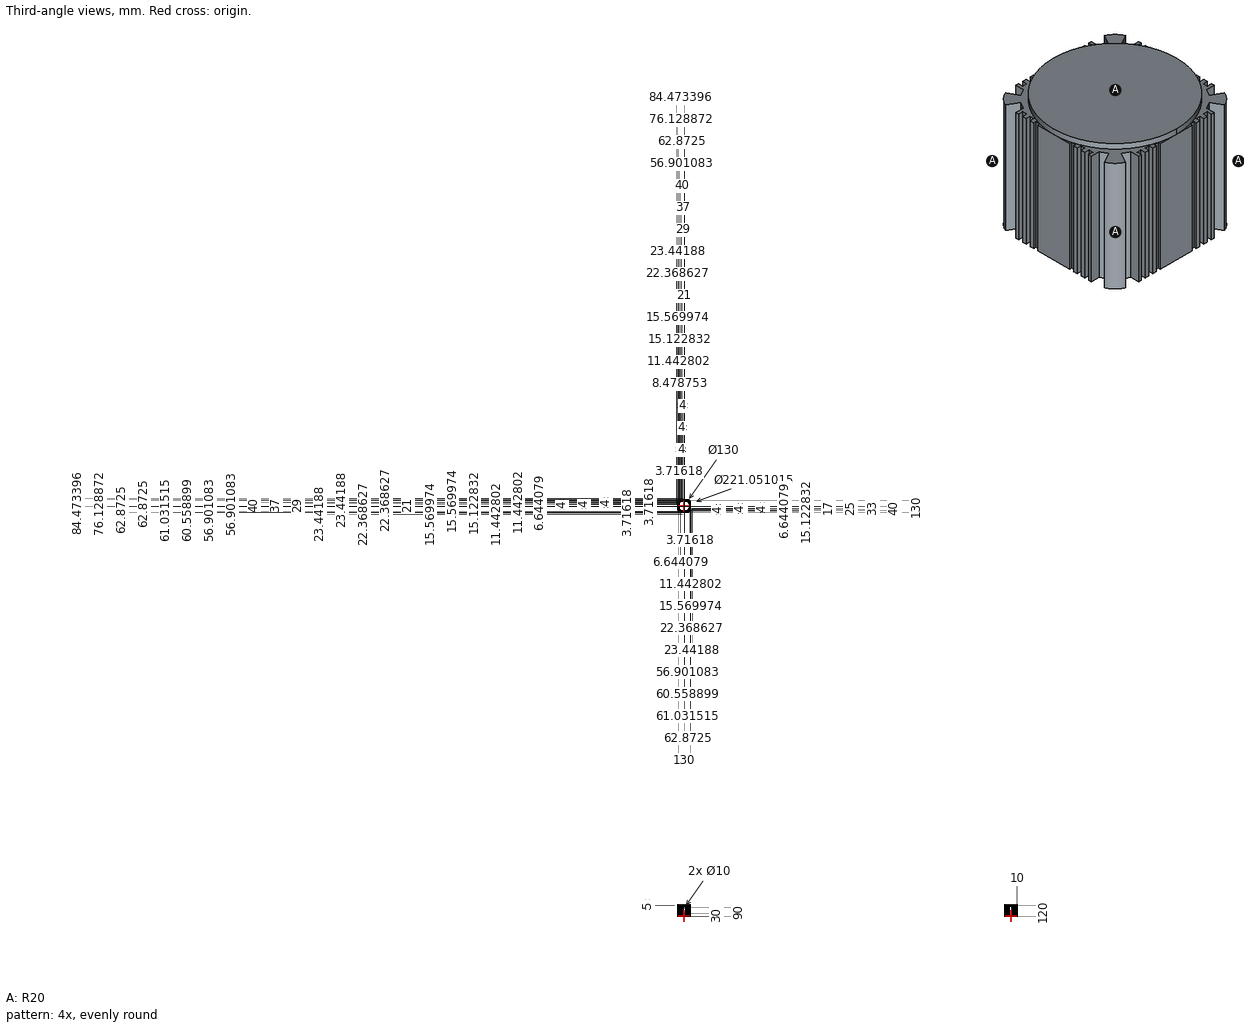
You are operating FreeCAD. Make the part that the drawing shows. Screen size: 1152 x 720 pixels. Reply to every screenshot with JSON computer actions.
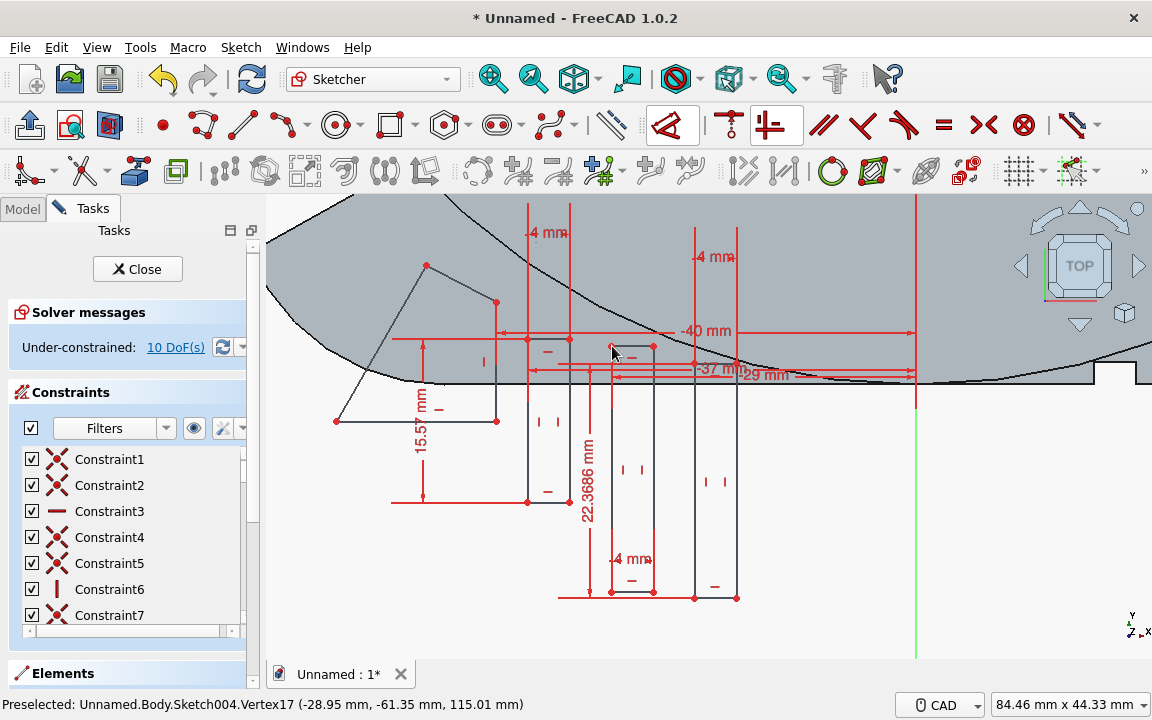
{"action": "left_click", "coordinate": [695, 364]}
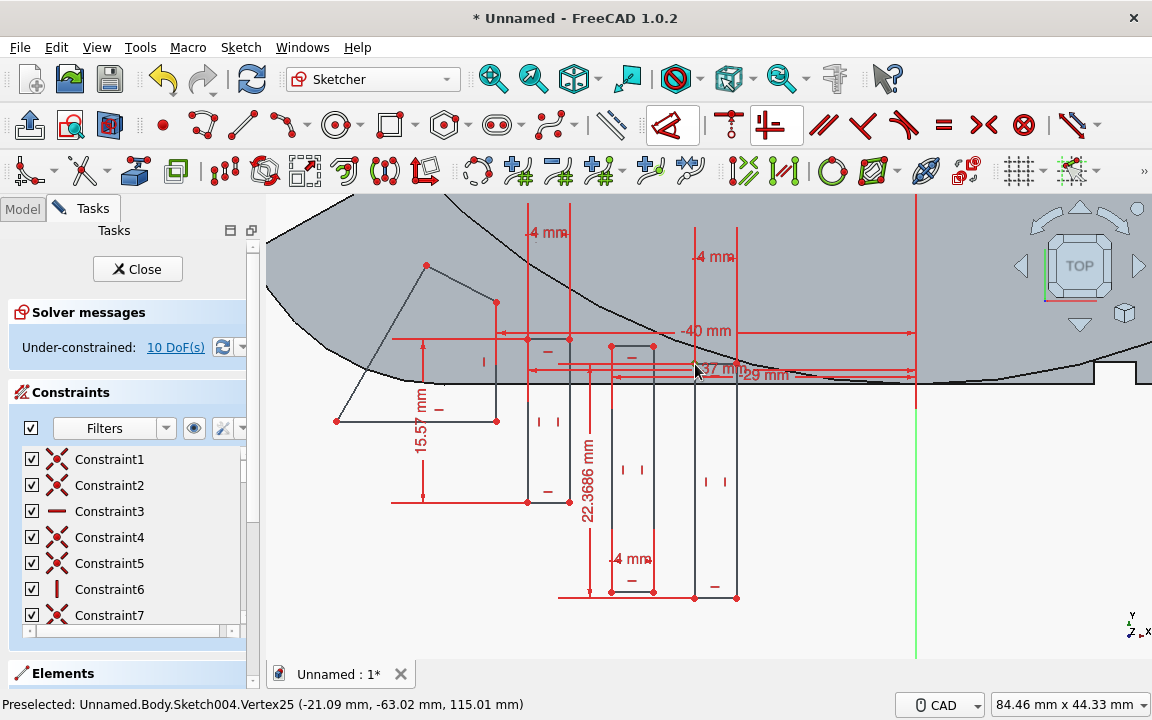
{"action": "key", "text": "l"}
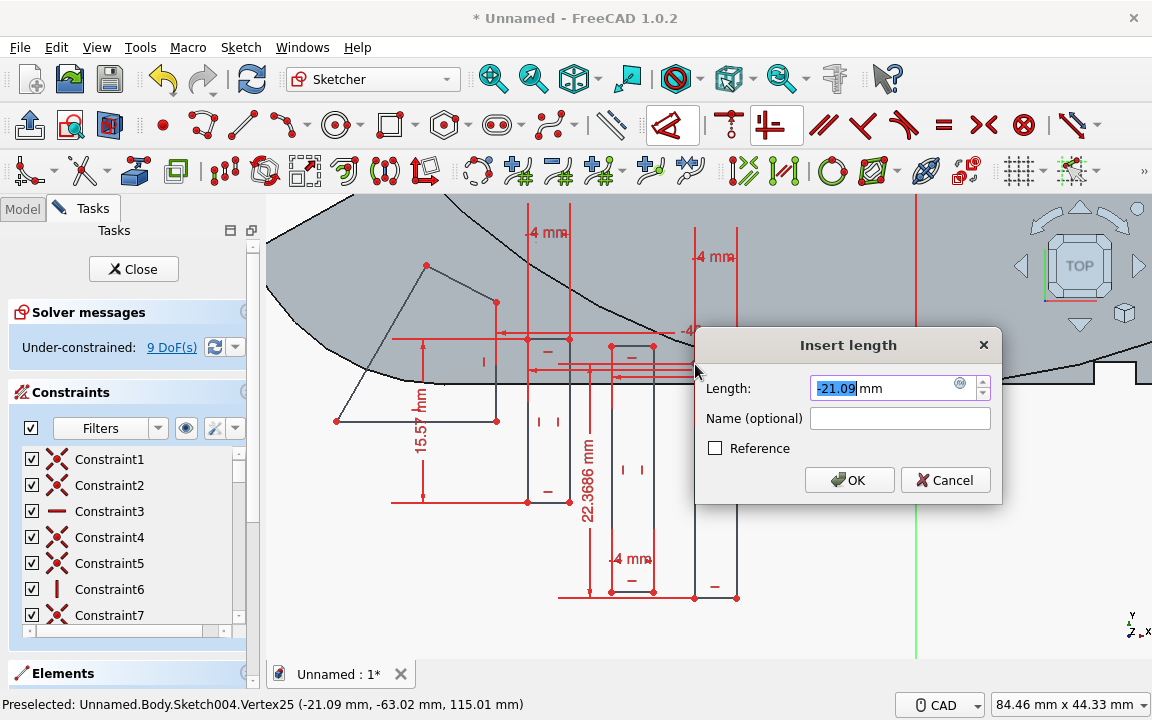
{"action": "type", "text": "-21"}
{"action": "key", "text": "Return"}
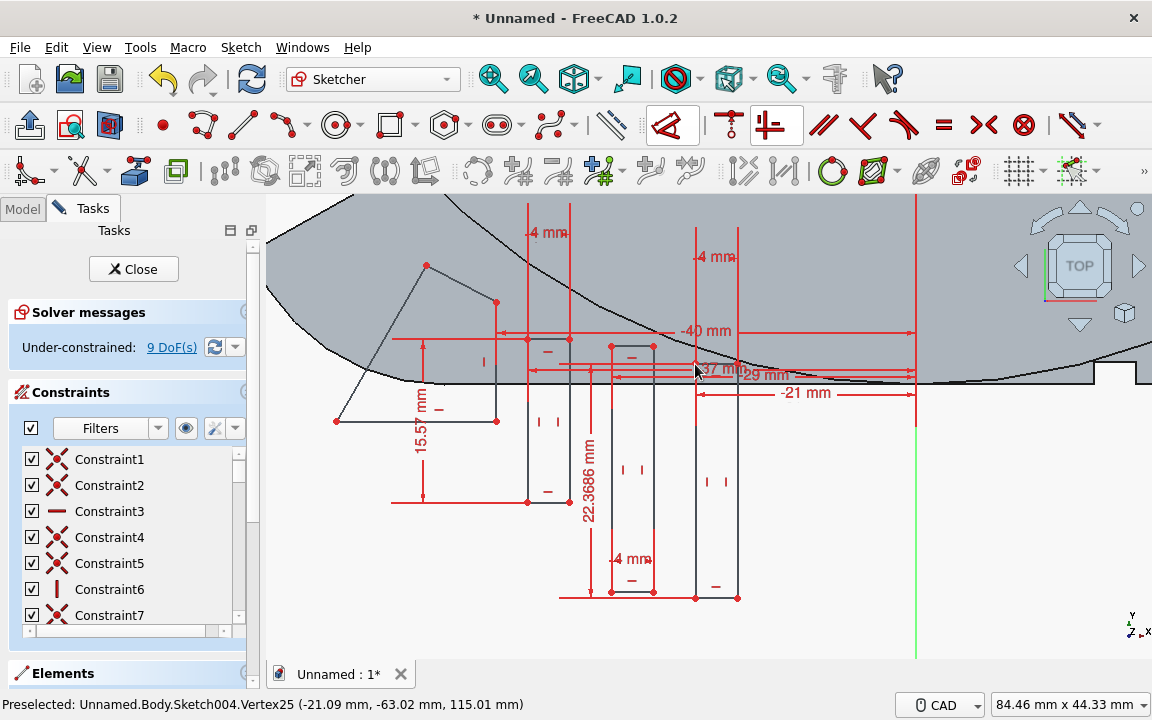
{"action": "left_click", "coordinate": [612, 420]}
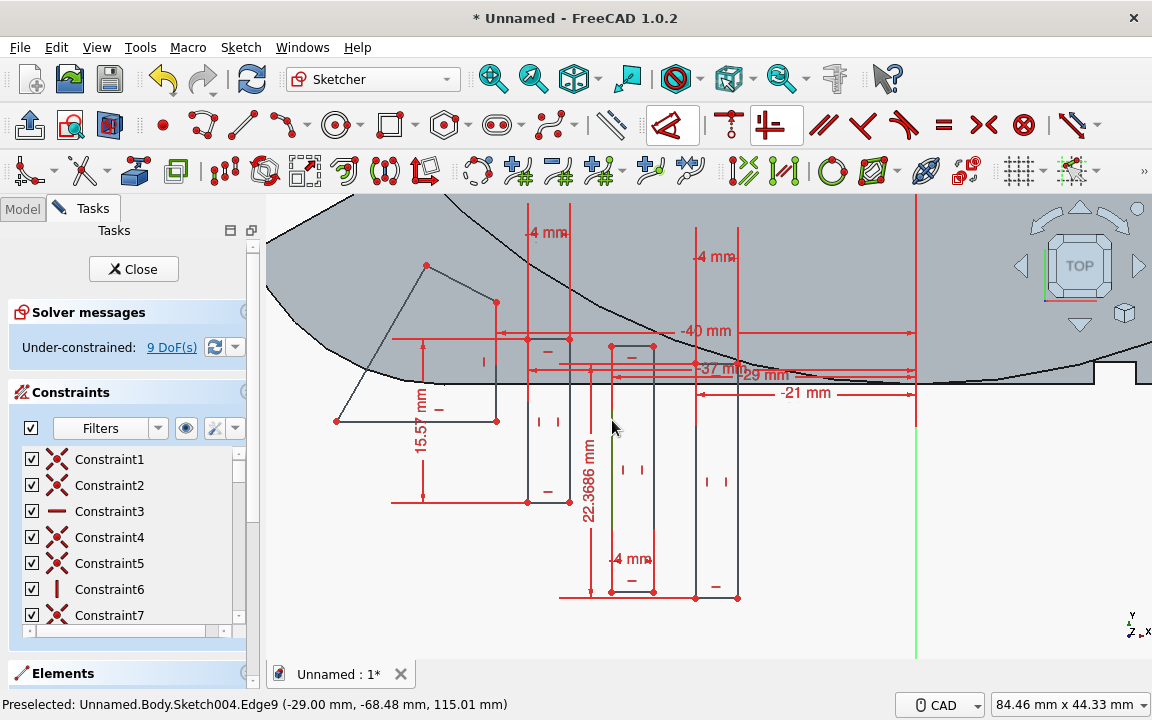
{"action": "key", "text": "i"}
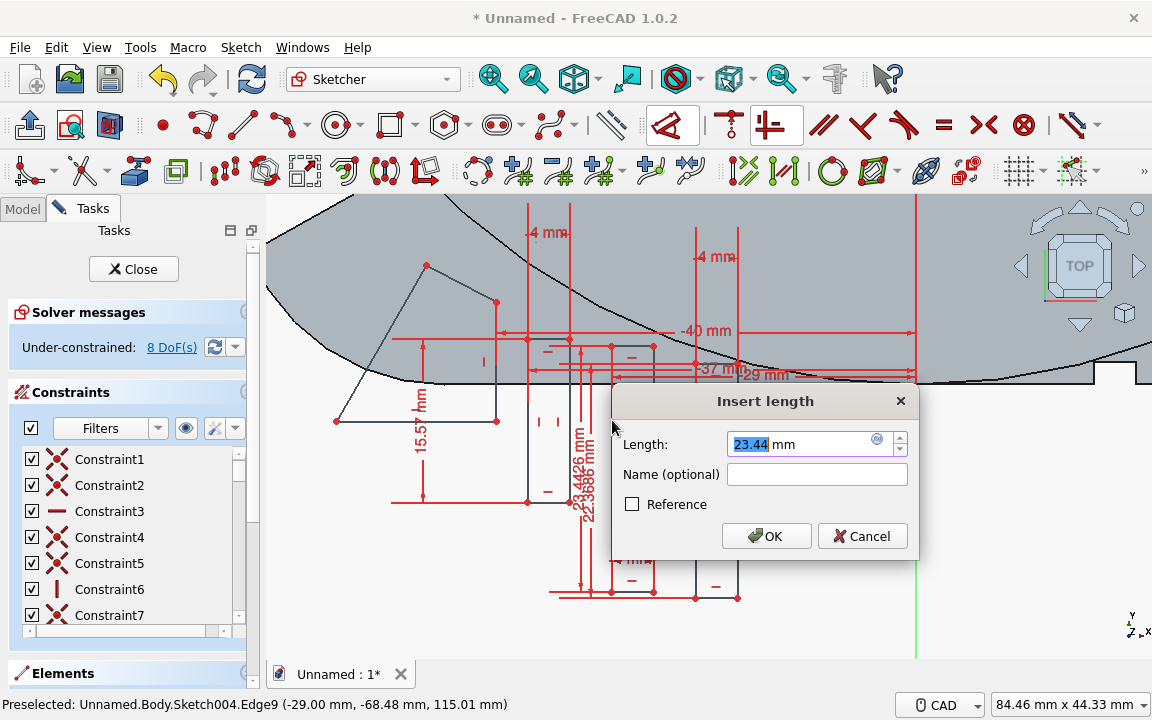
{"action": "type", "text": "23.44188"}
{"action": "key", "text": "Return"}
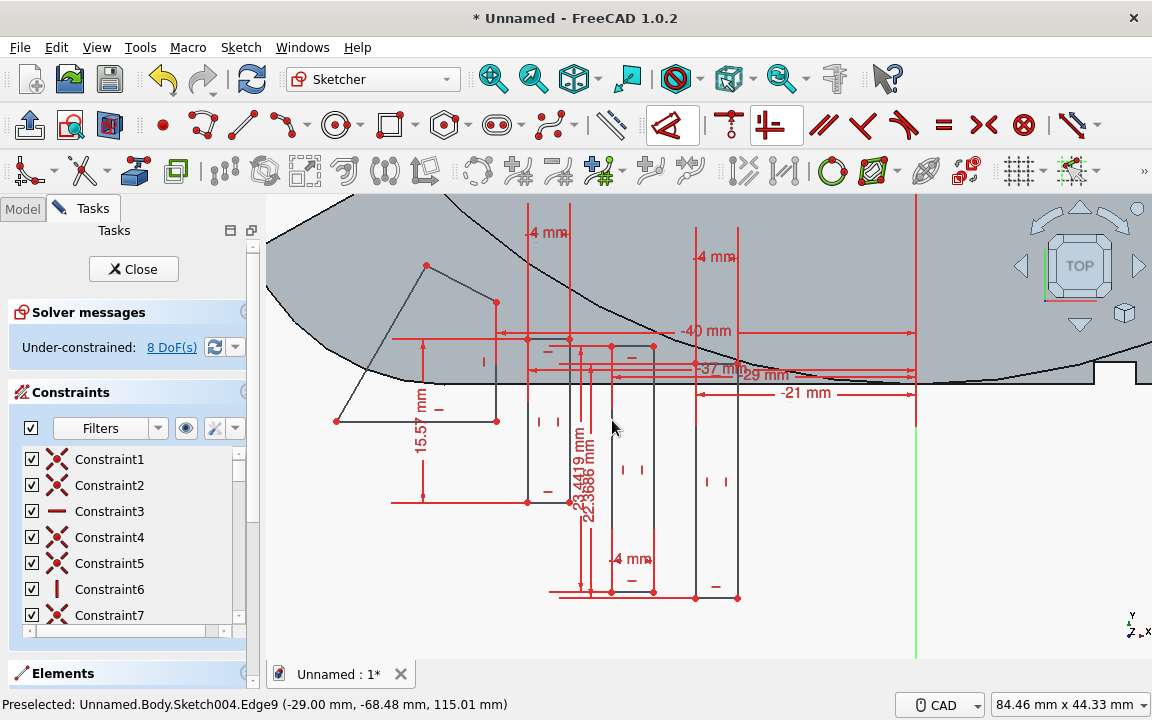
{"action": "left_click", "coordinate": [696, 364]}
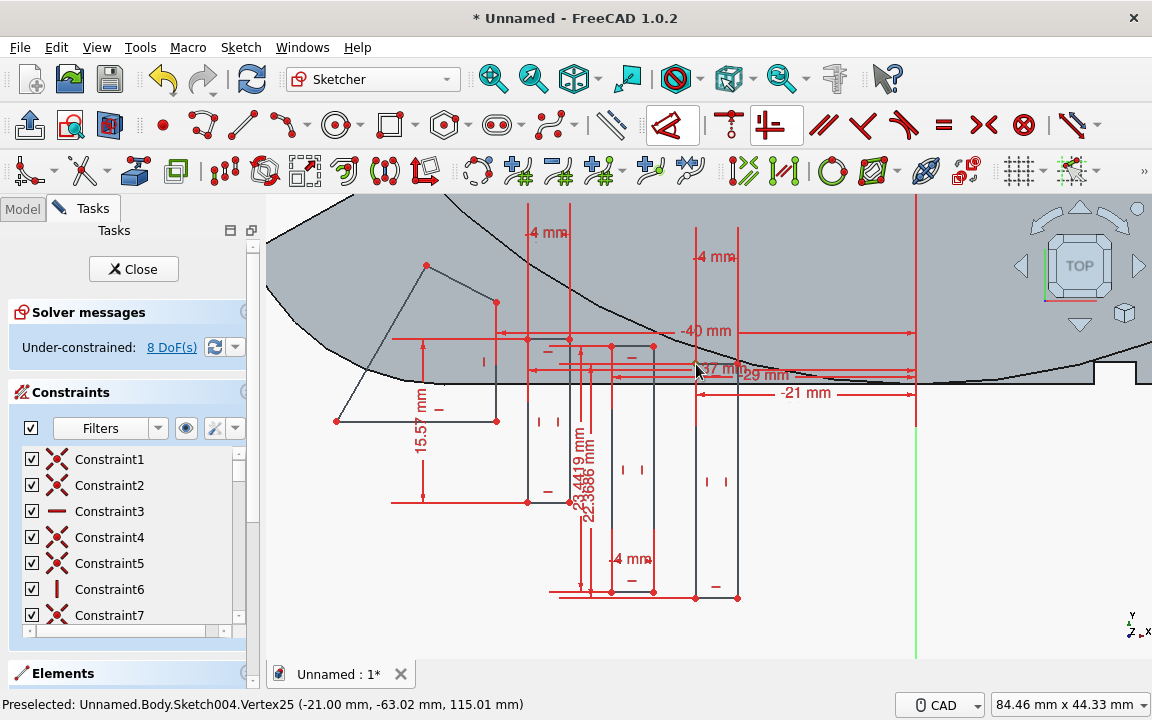
{"action": "key", "text": "i"}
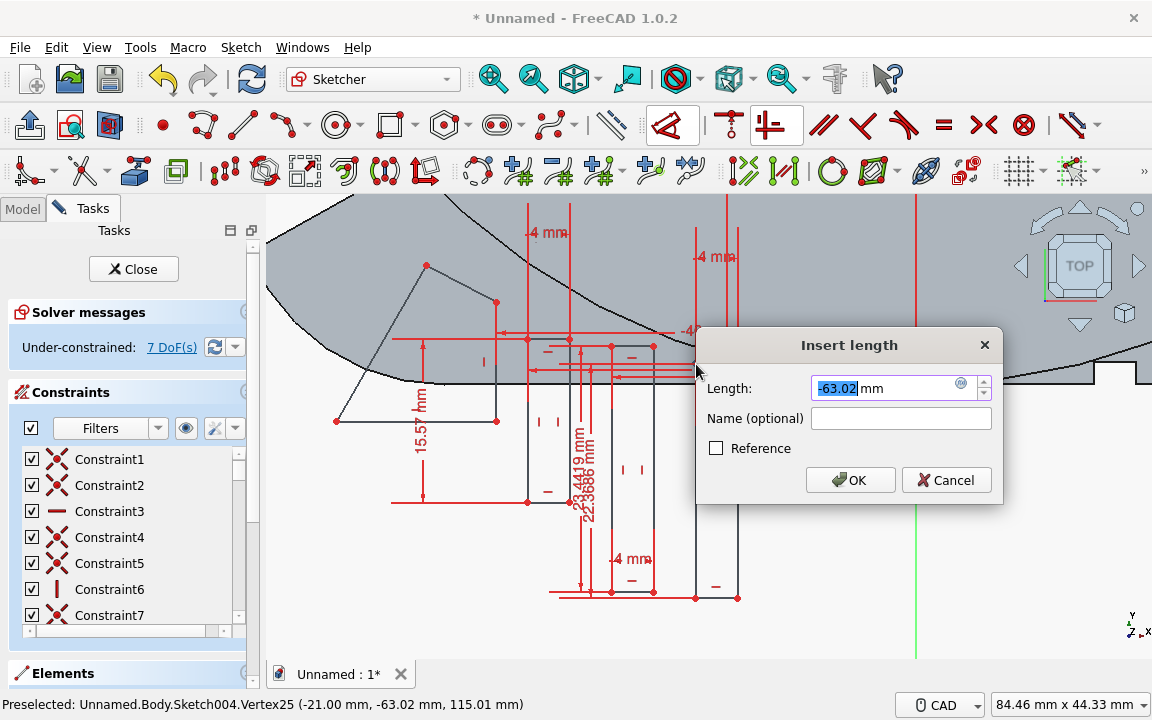
{"action": "type", "text": "-62.8725"}
{"action": "key", "text": "Return"}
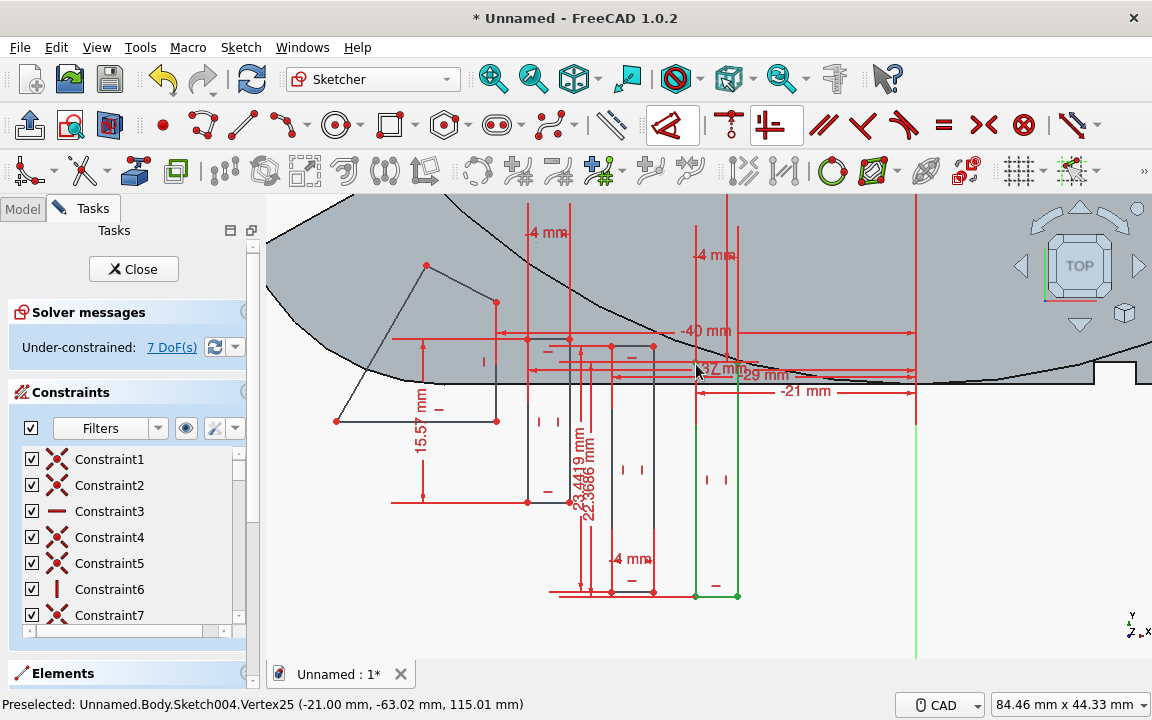
{"action": "left_click", "coordinate": [475, 291]}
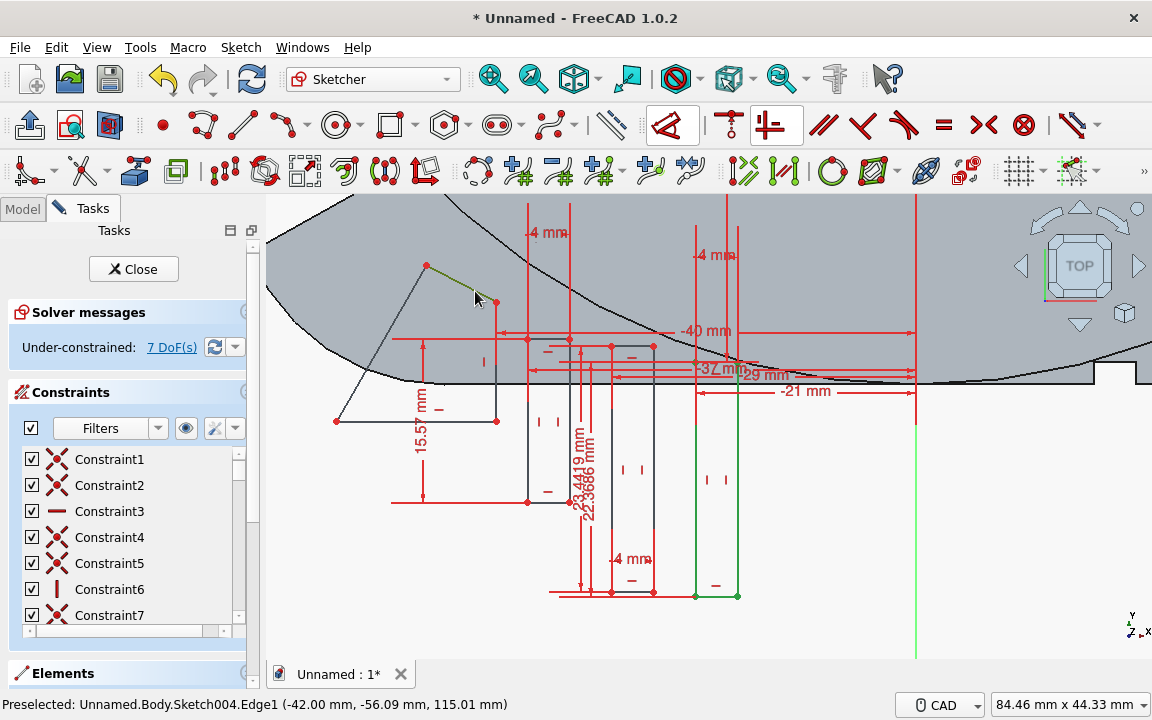
{"action": "key", "text": "i"}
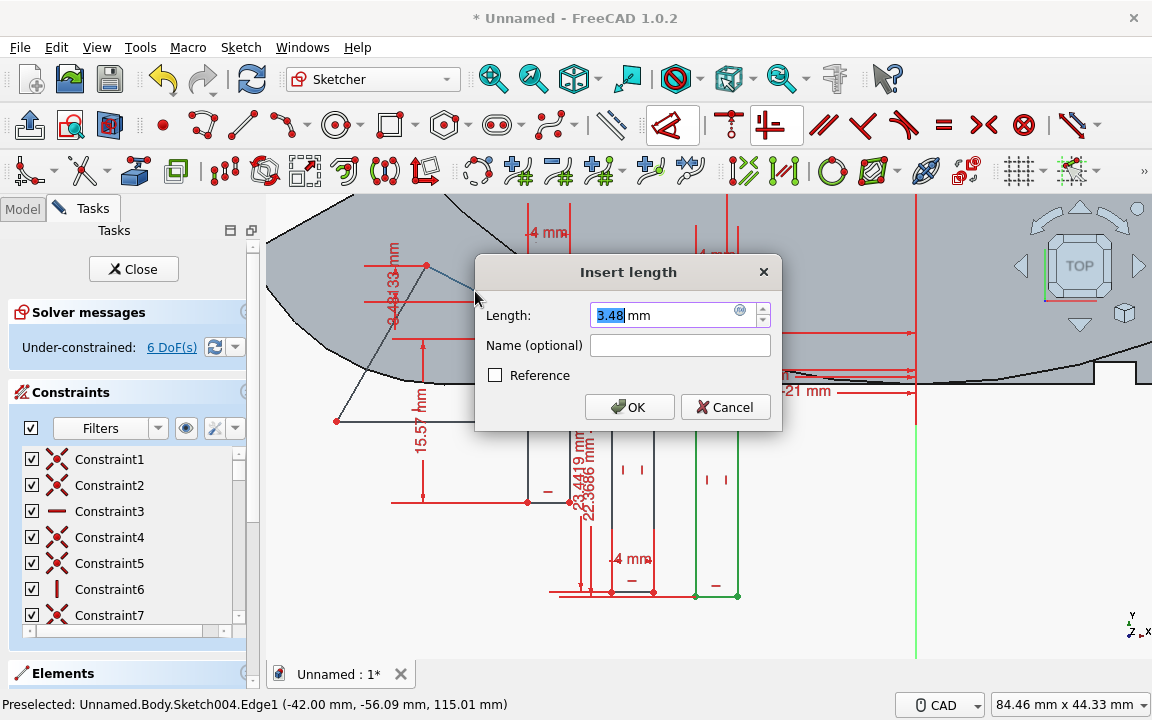
{"action": "type", "text": "3.71618"}
{"action": "key", "text": "Return"}